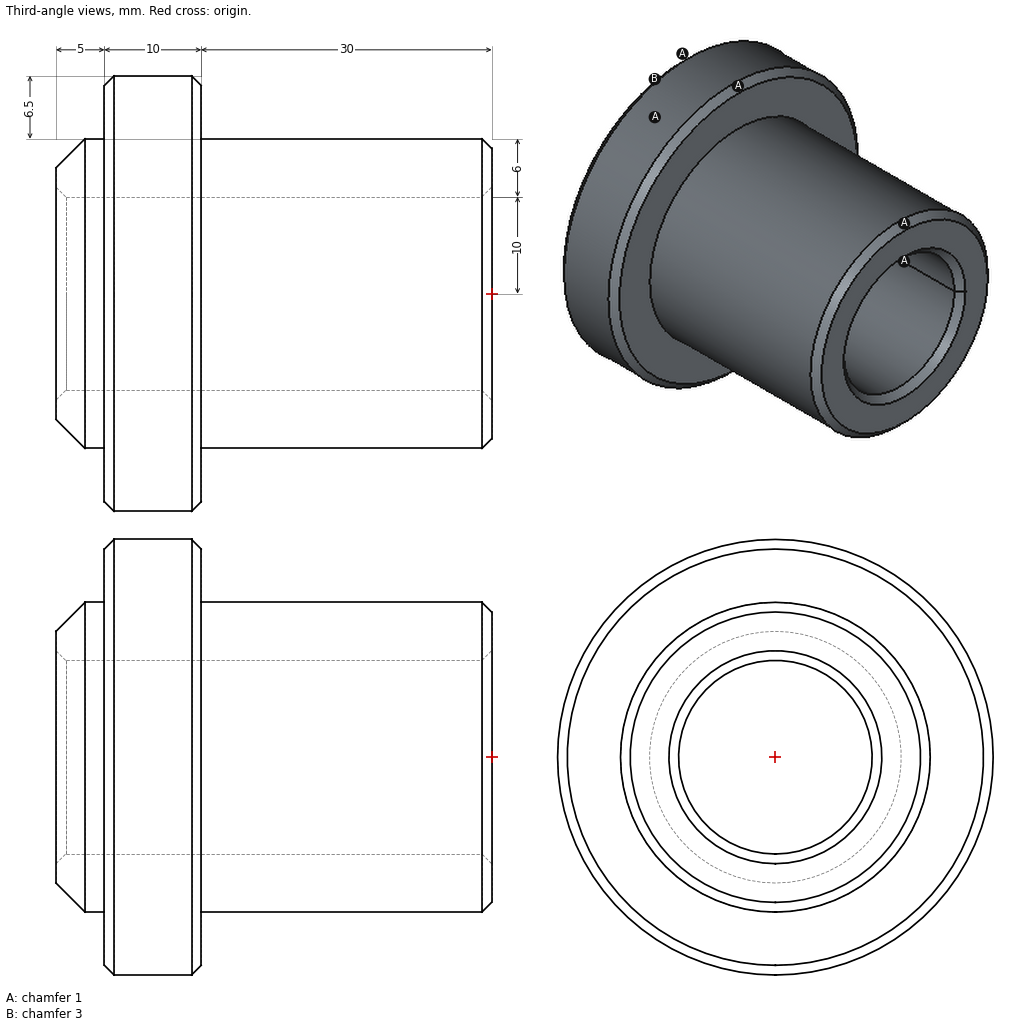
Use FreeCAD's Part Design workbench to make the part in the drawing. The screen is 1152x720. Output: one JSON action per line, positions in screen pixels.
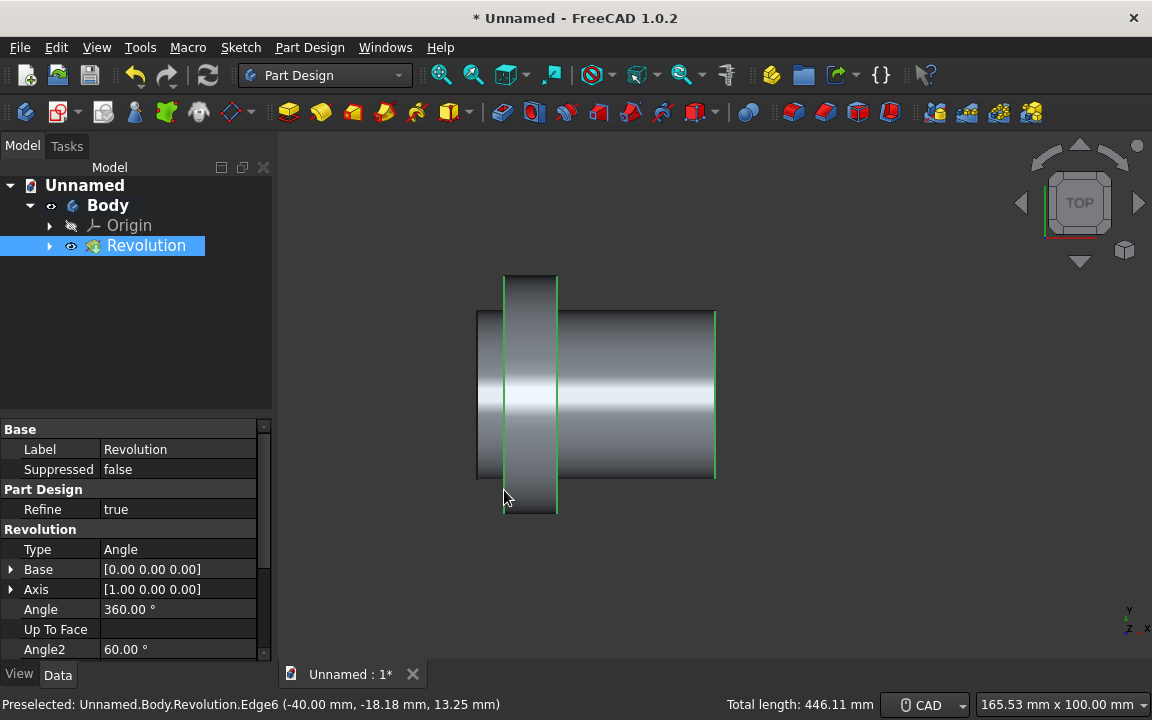
{"action": "key", "text": "1"}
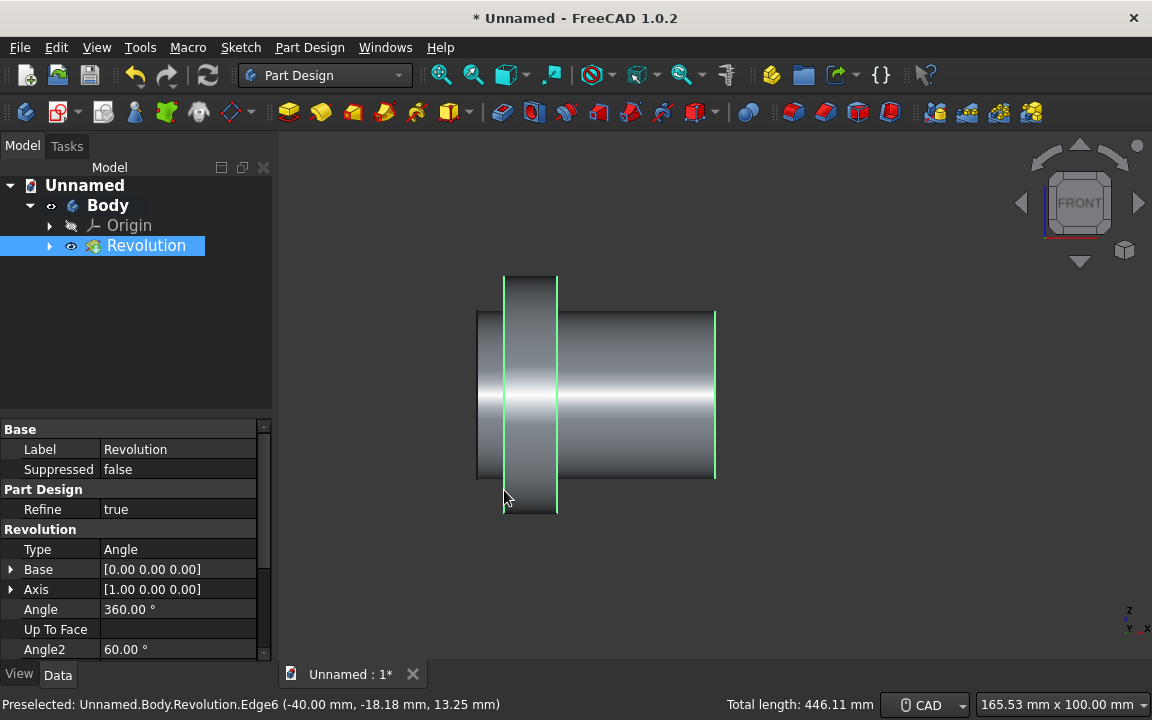
{"action": "key", "text": "3"}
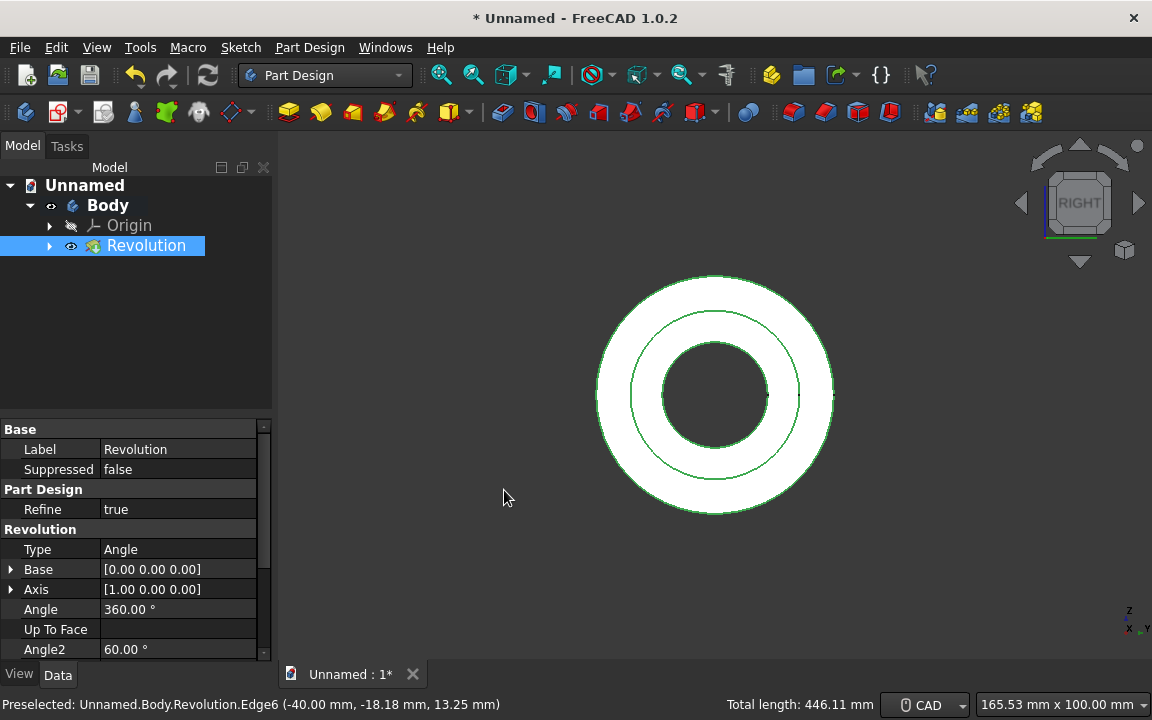
{"action": "key", "text": "5"}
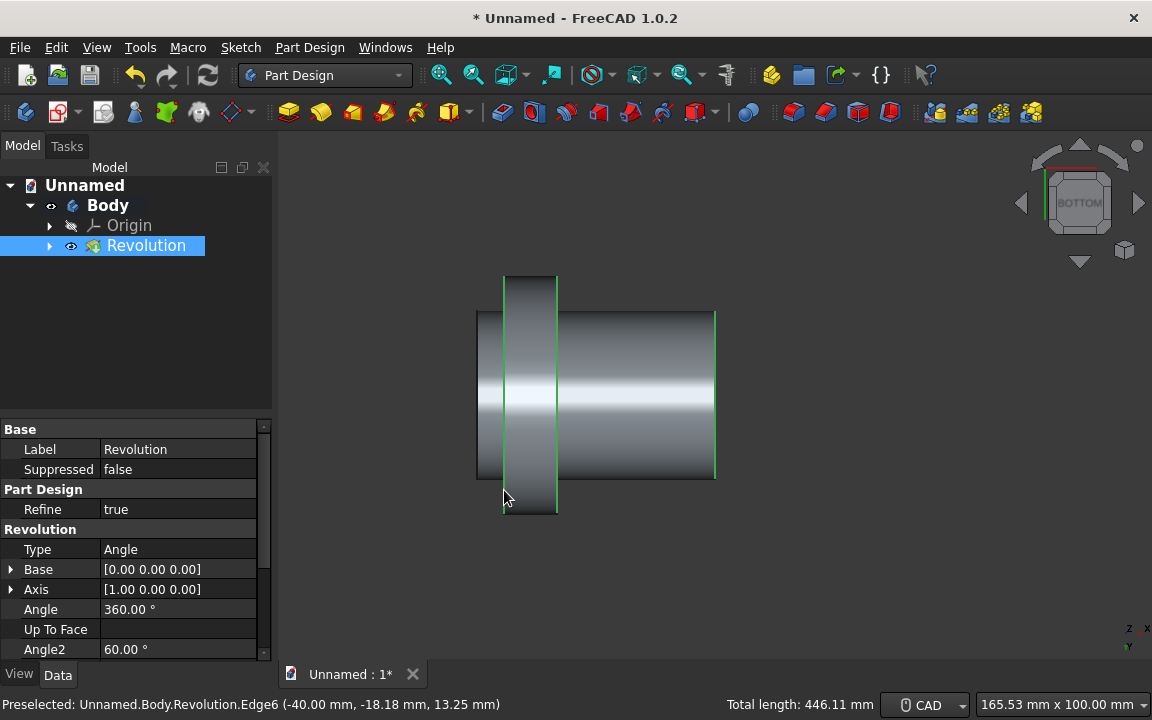
{"action": "key", "text": "4"}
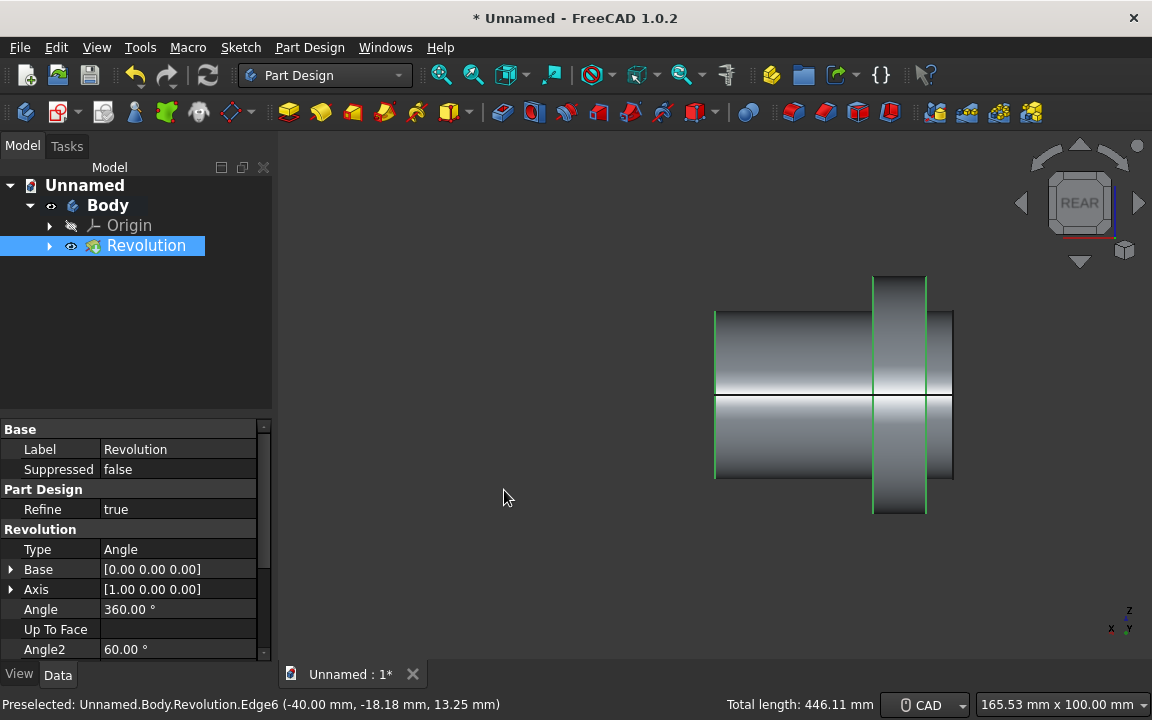
{"action": "key", "text": "6"}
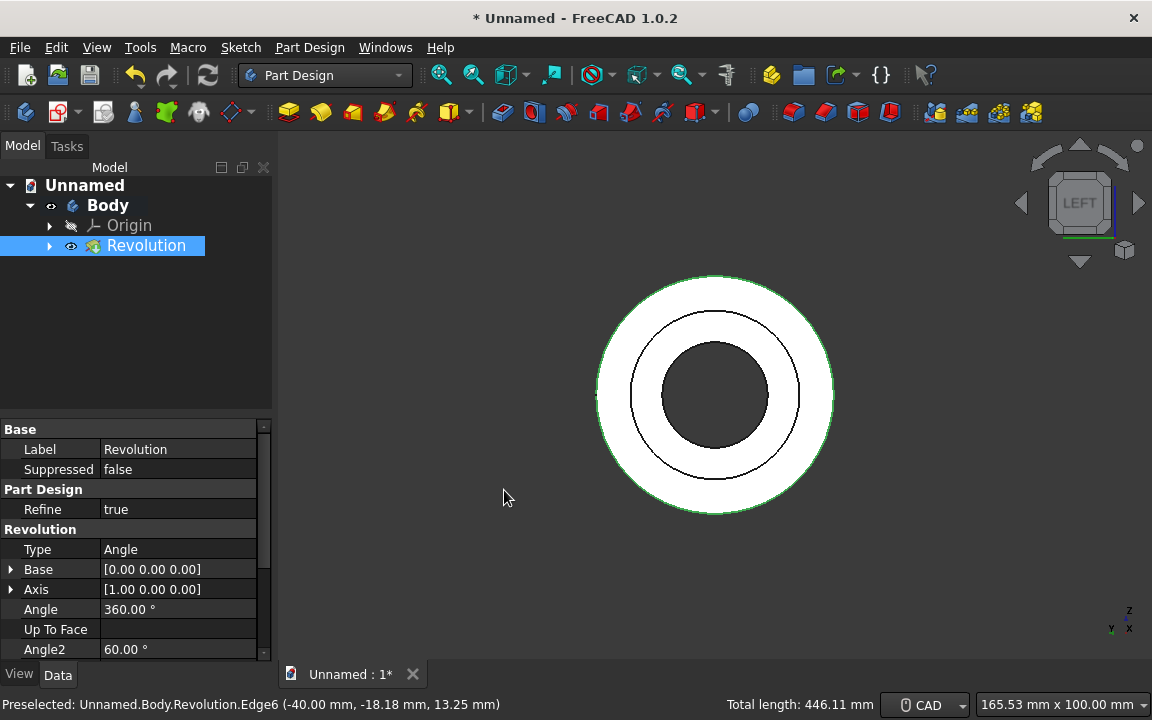
{"action": "left_click", "coordinate": [768, 394], "text": "ctrl"}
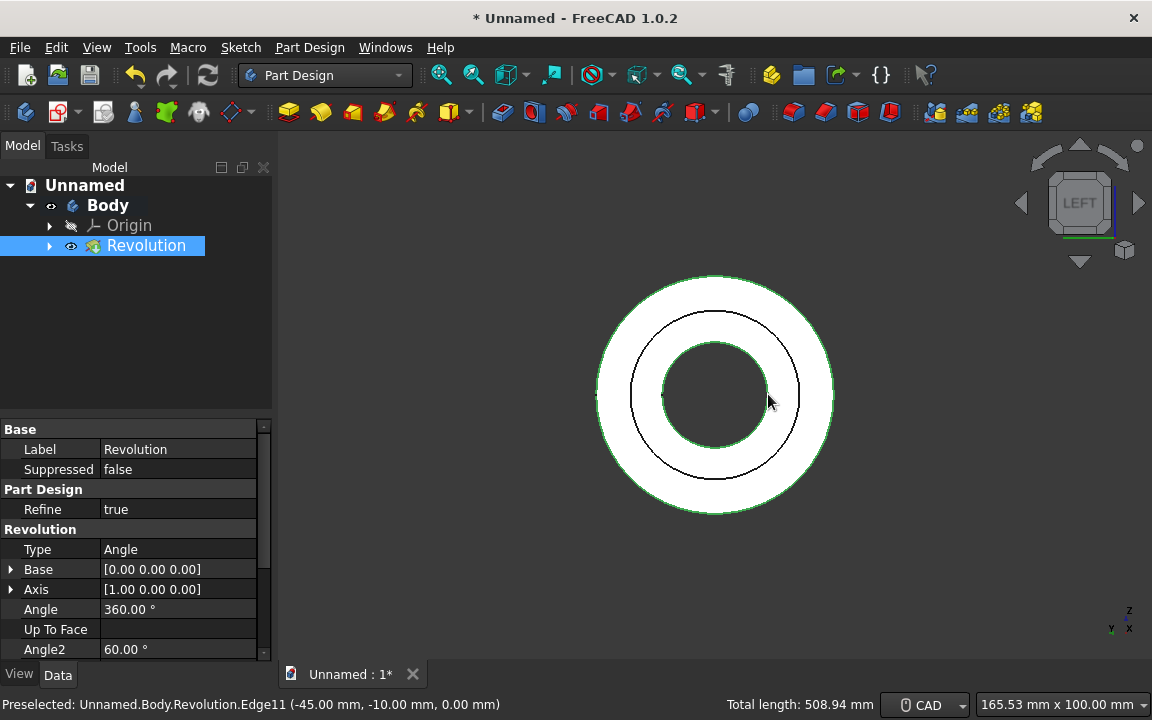
{"action": "left_click", "coordinate": [826, 112]}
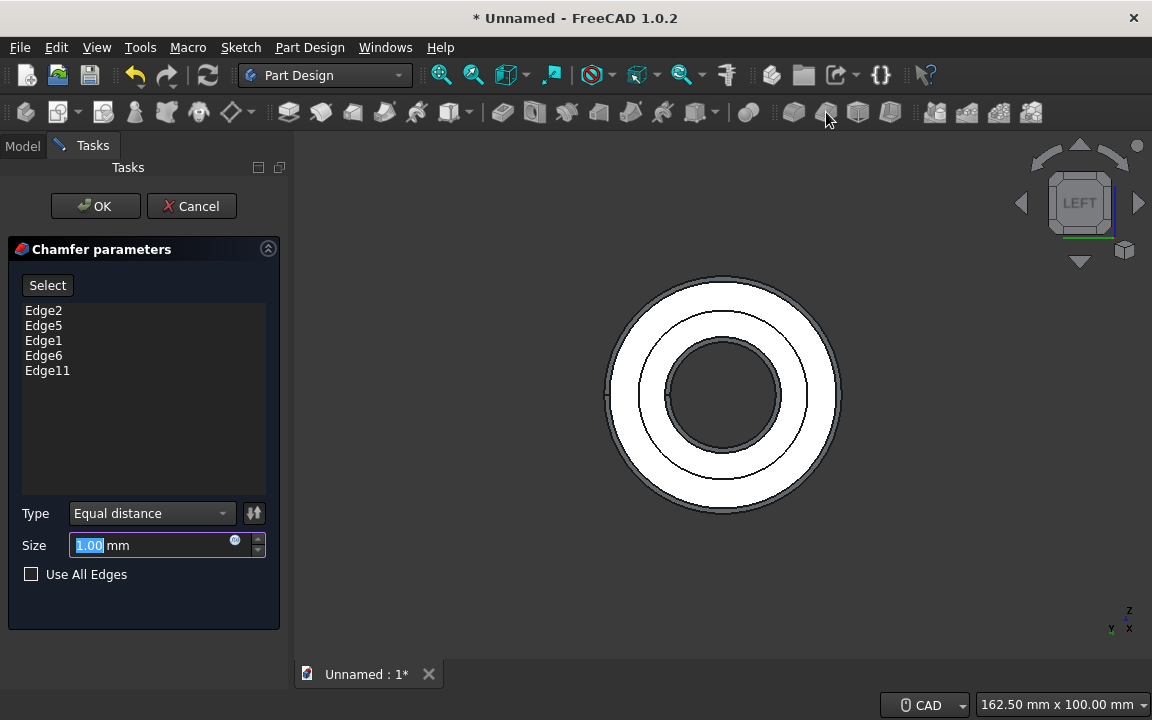
{"action": "type", "text": "1"}
{"action": "key", "text": "Tab"}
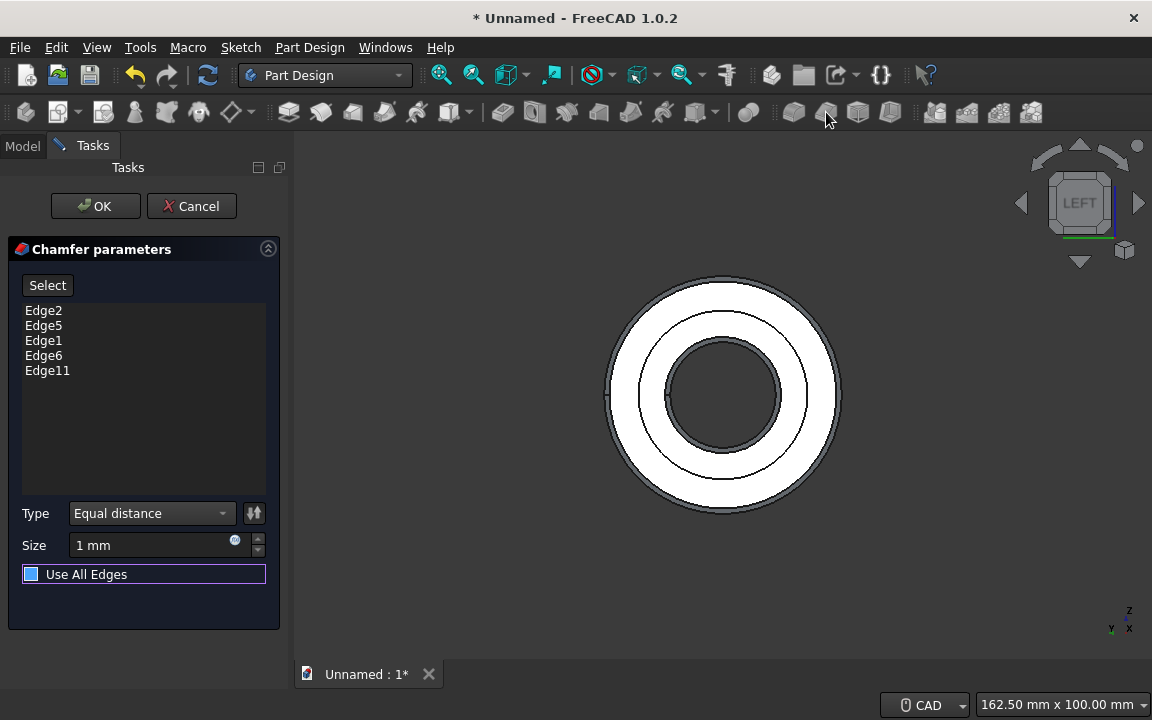
{"action": "left_click", "coordinate": [96, 206]}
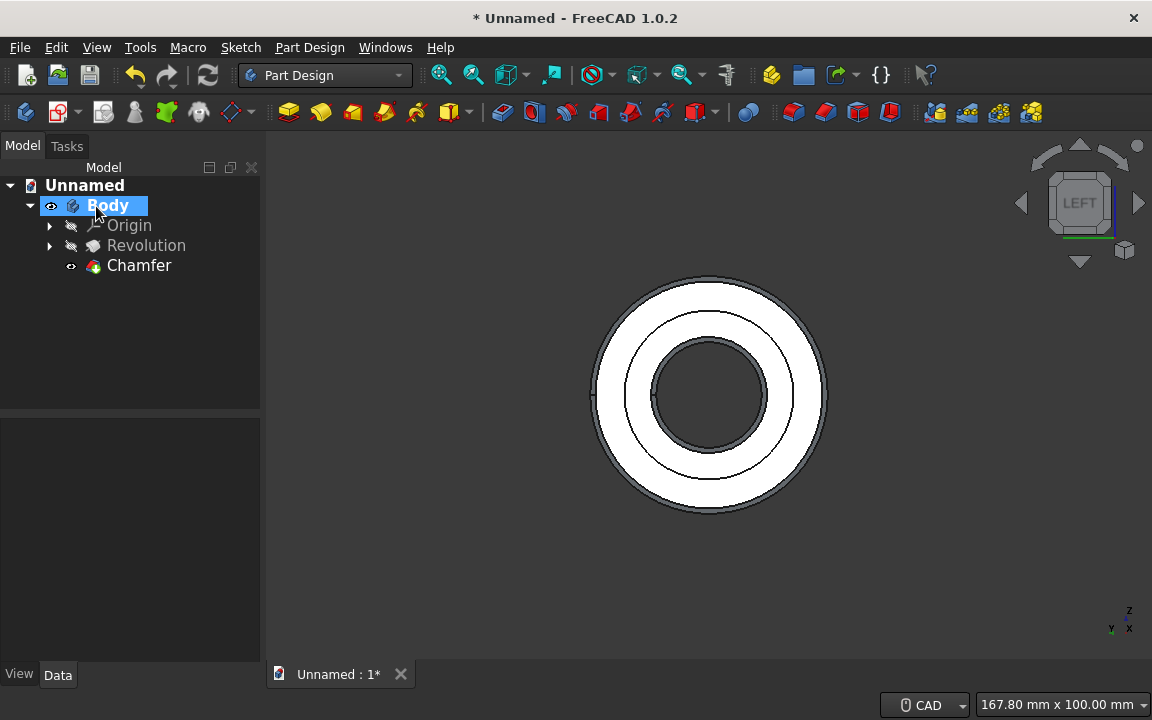
{"action": "left_click", "coordinate": [793, 394]}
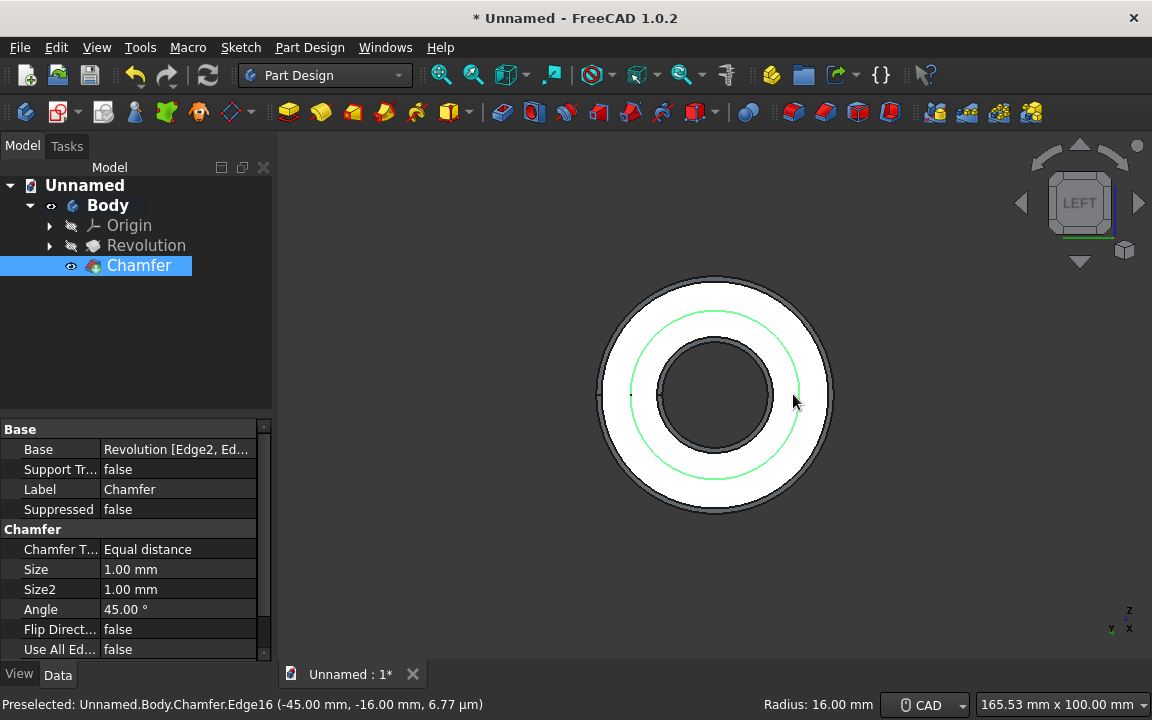
{"action": "left_click", "coordinate": [826, 112]}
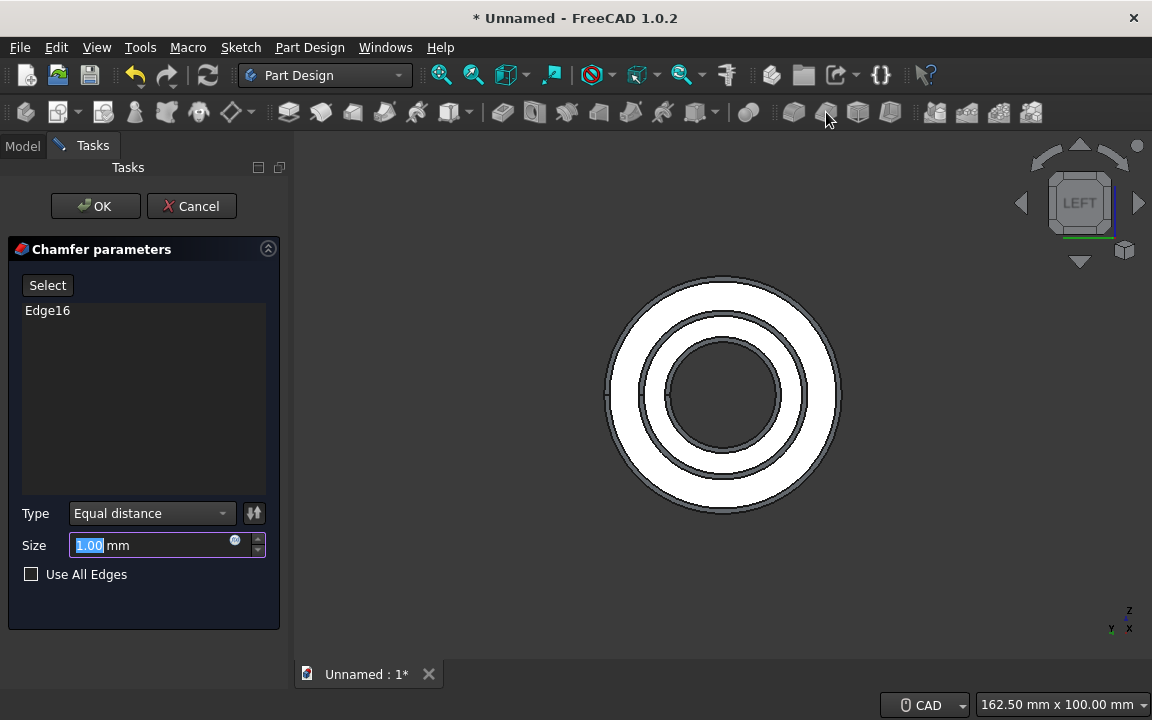
{"action": "type", "text": "3"}
{"action": "key", "text": "Tab"}